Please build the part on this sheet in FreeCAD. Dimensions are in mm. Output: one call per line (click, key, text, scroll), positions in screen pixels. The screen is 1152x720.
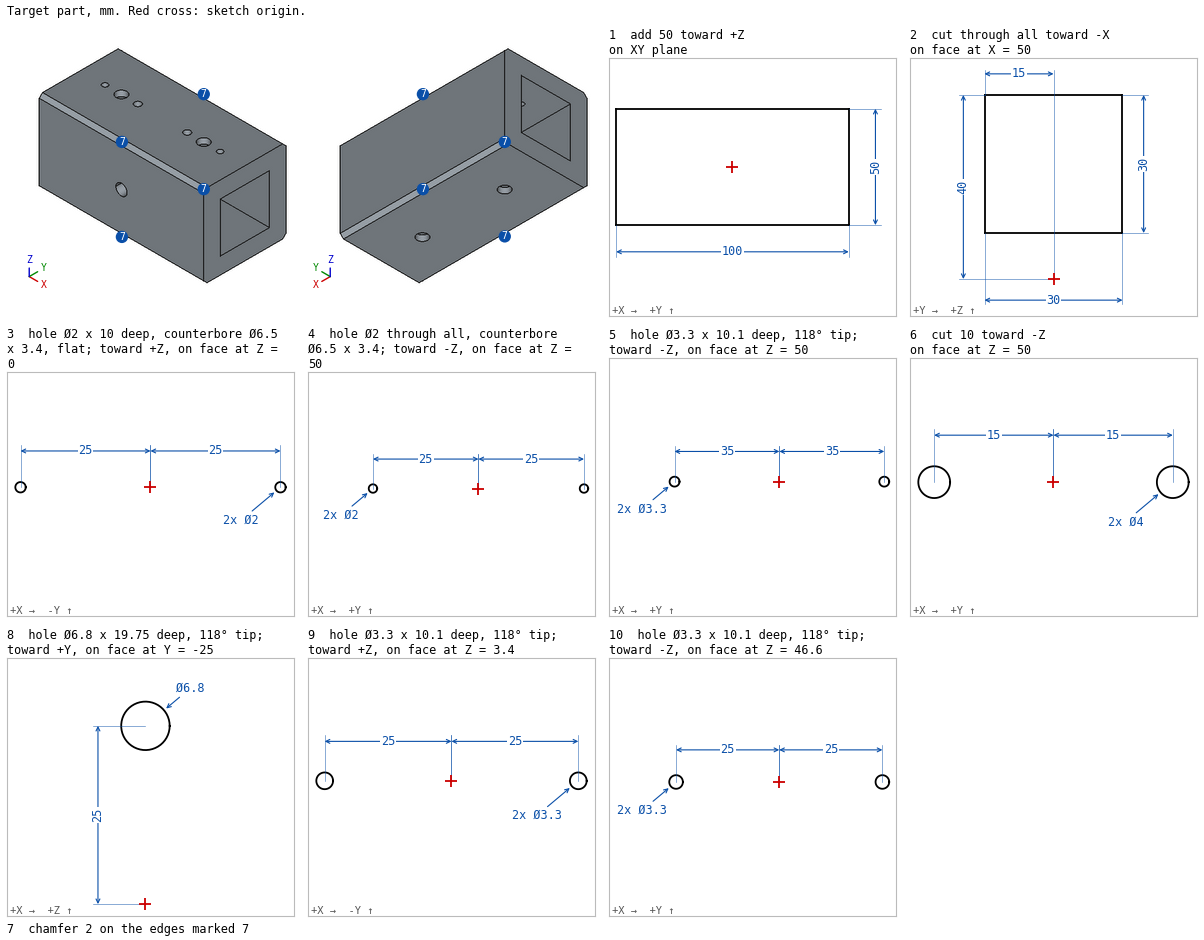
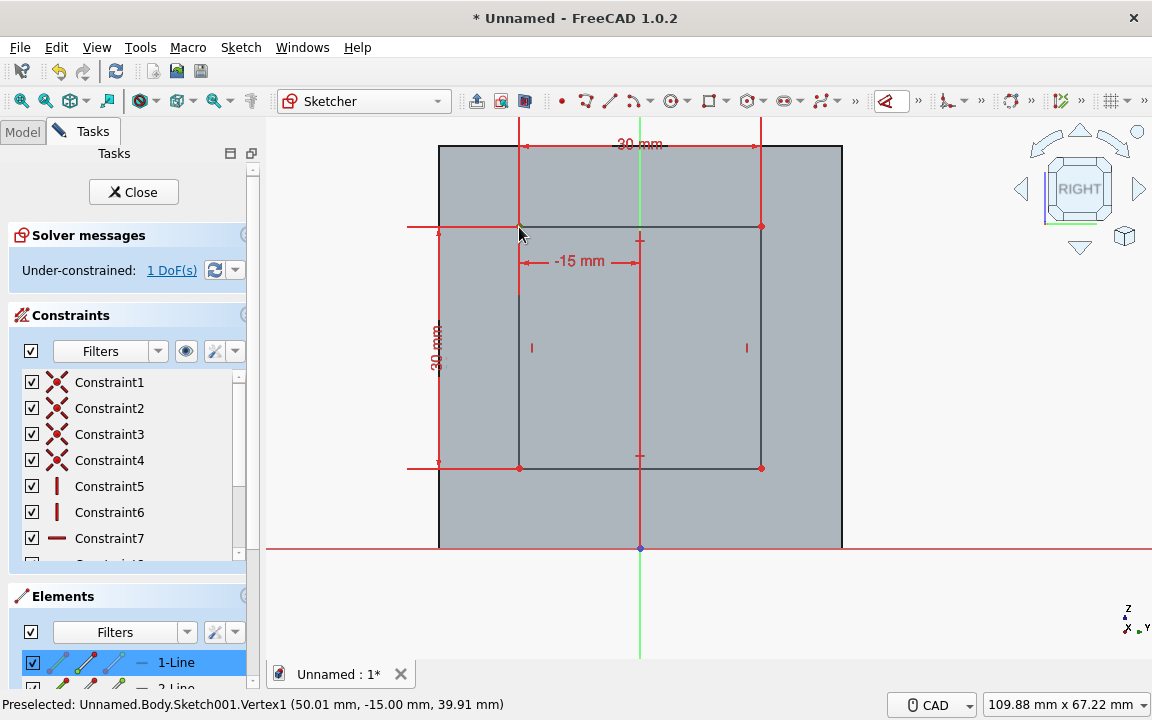
click(904, 102)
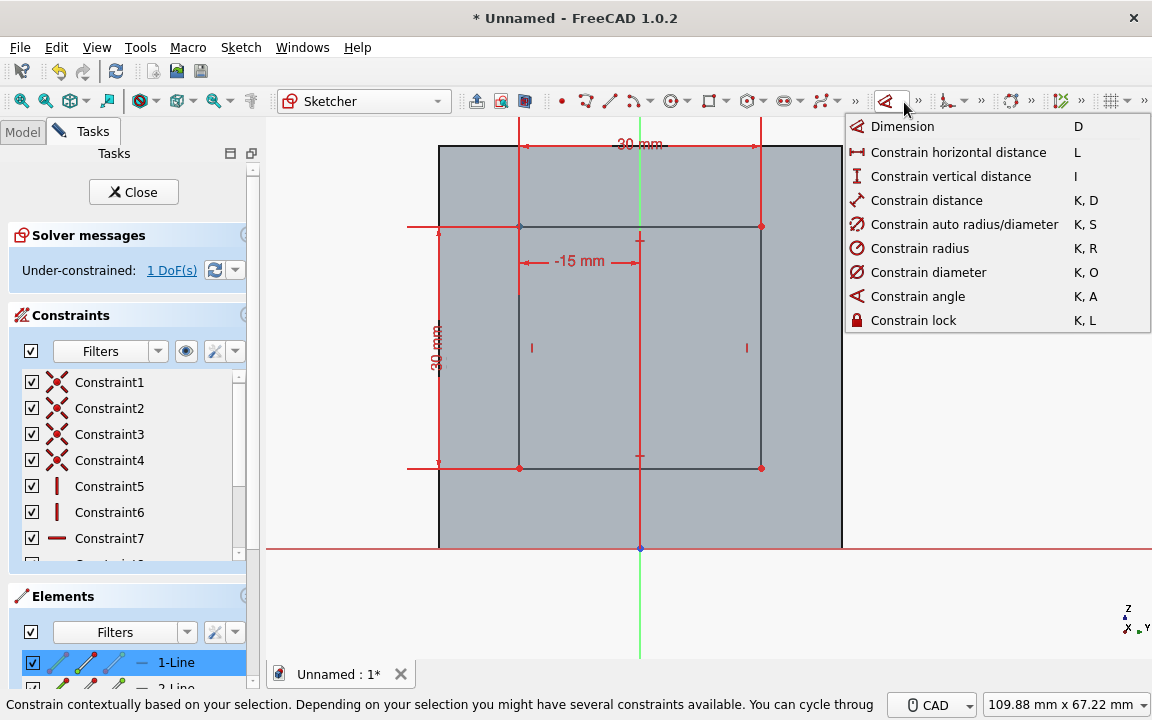
click(998, 176)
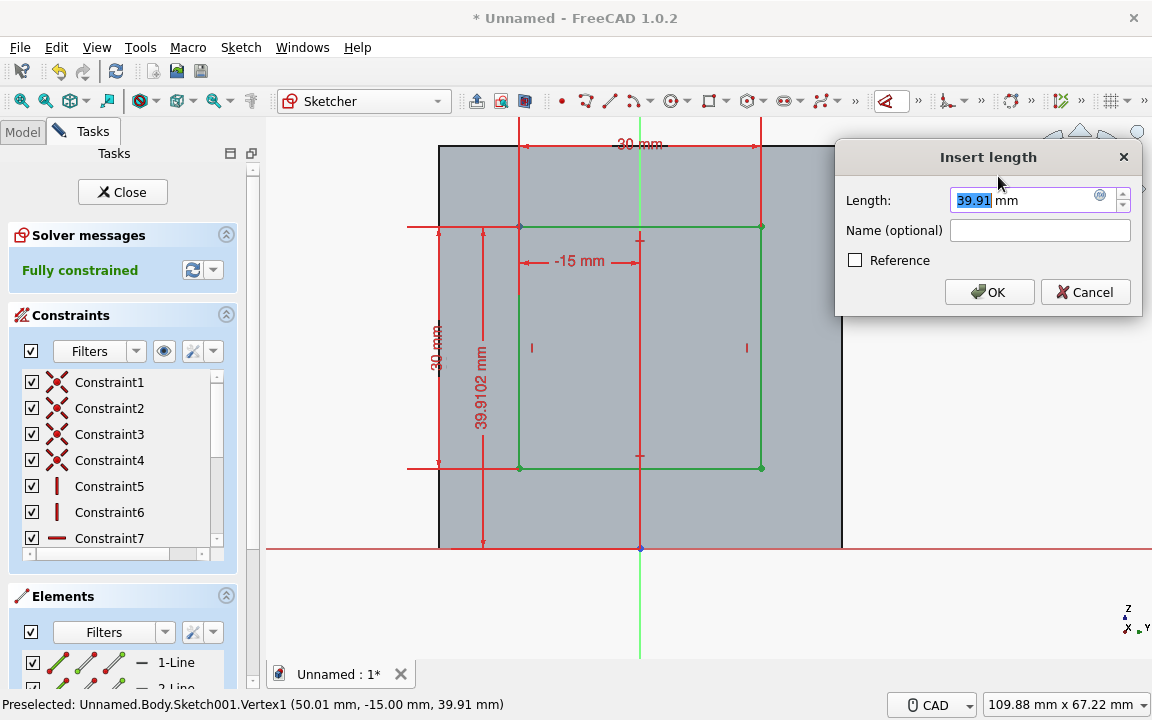
text(40)
key(Return)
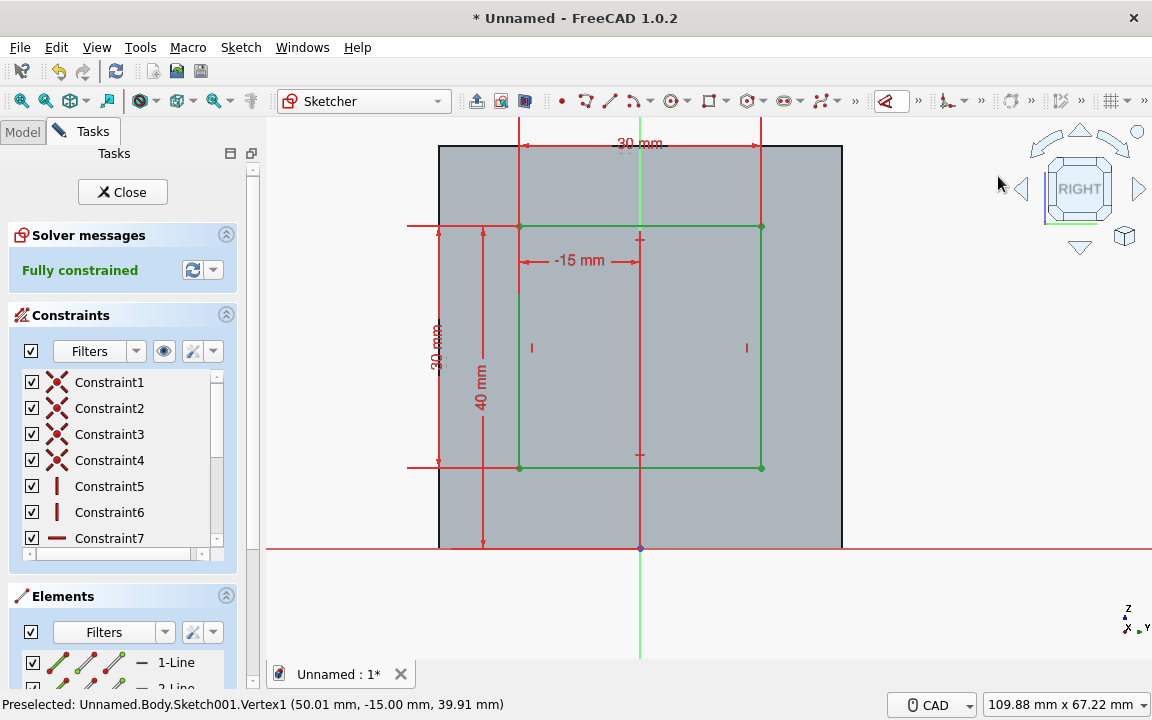
click(123, 192)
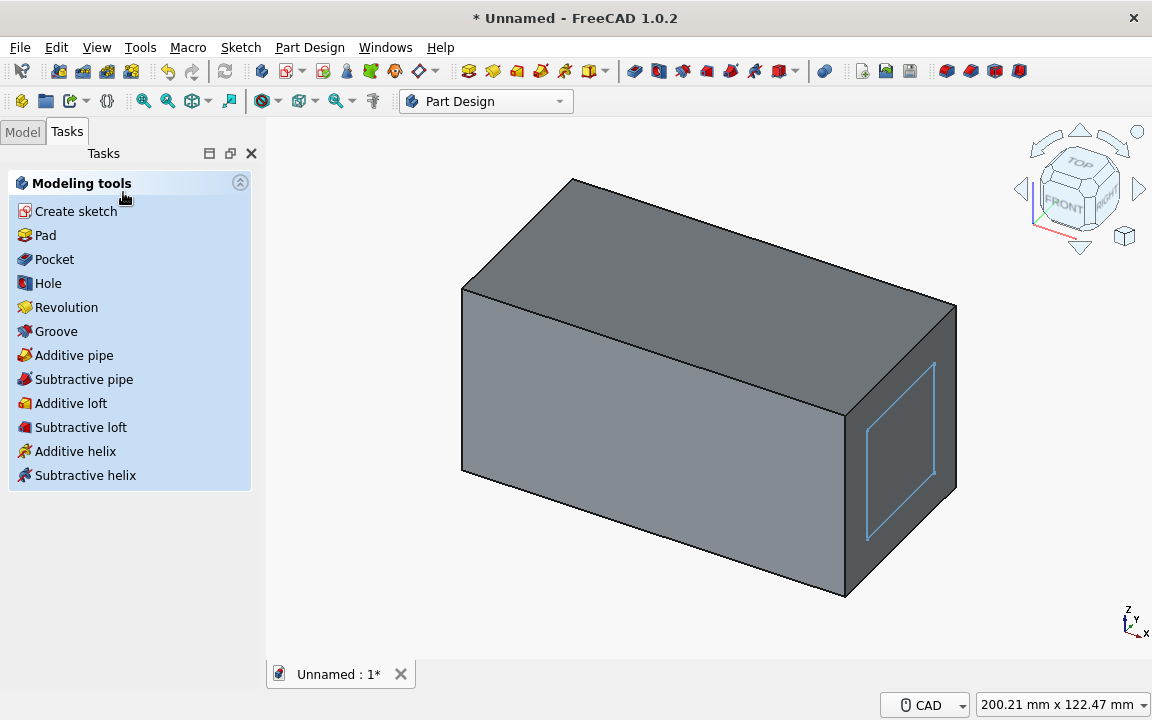
click(636, 72)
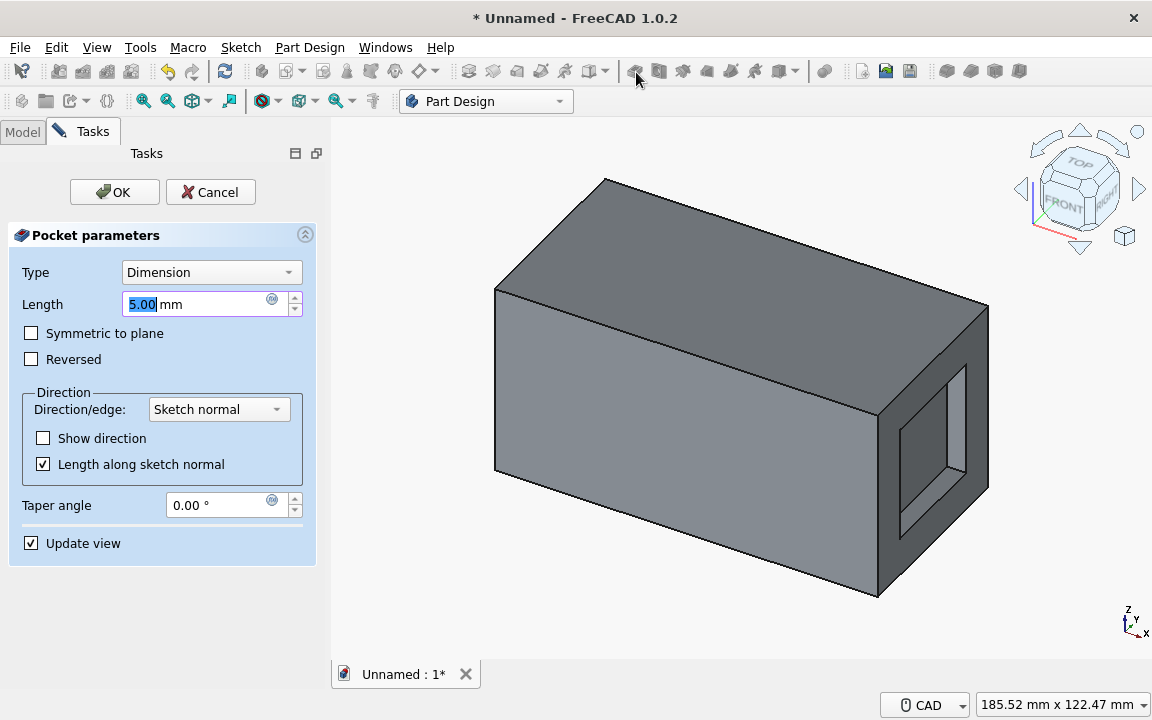
click(212, 272)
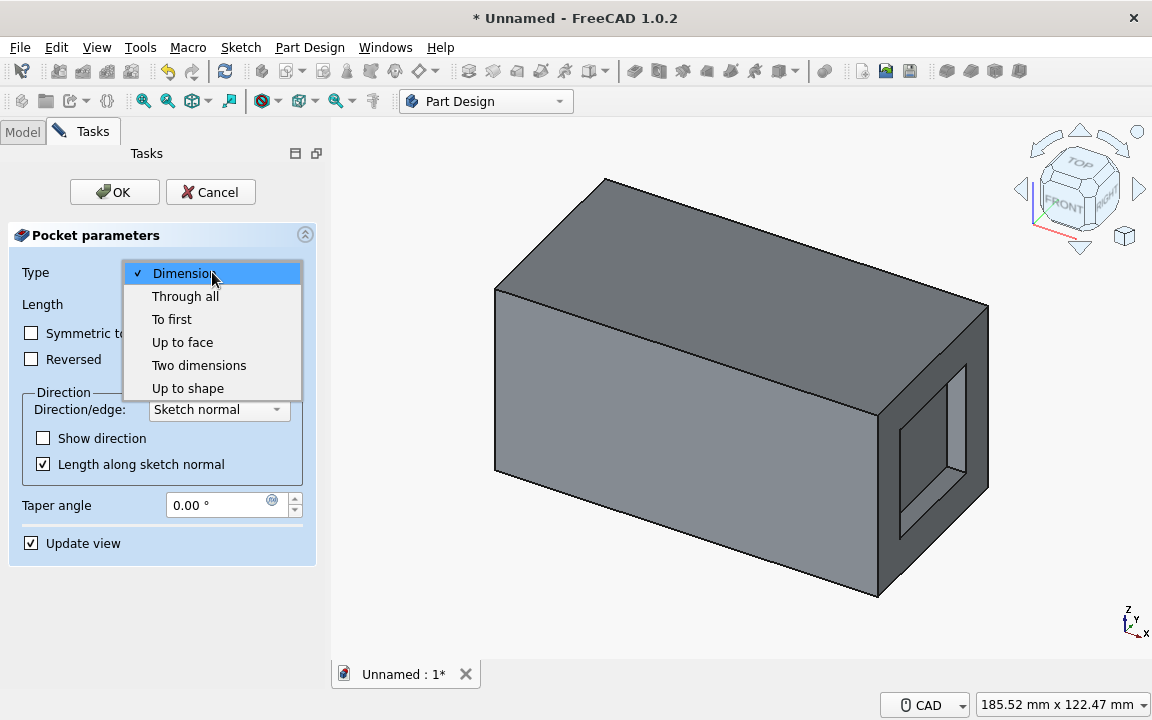
click(212, 296)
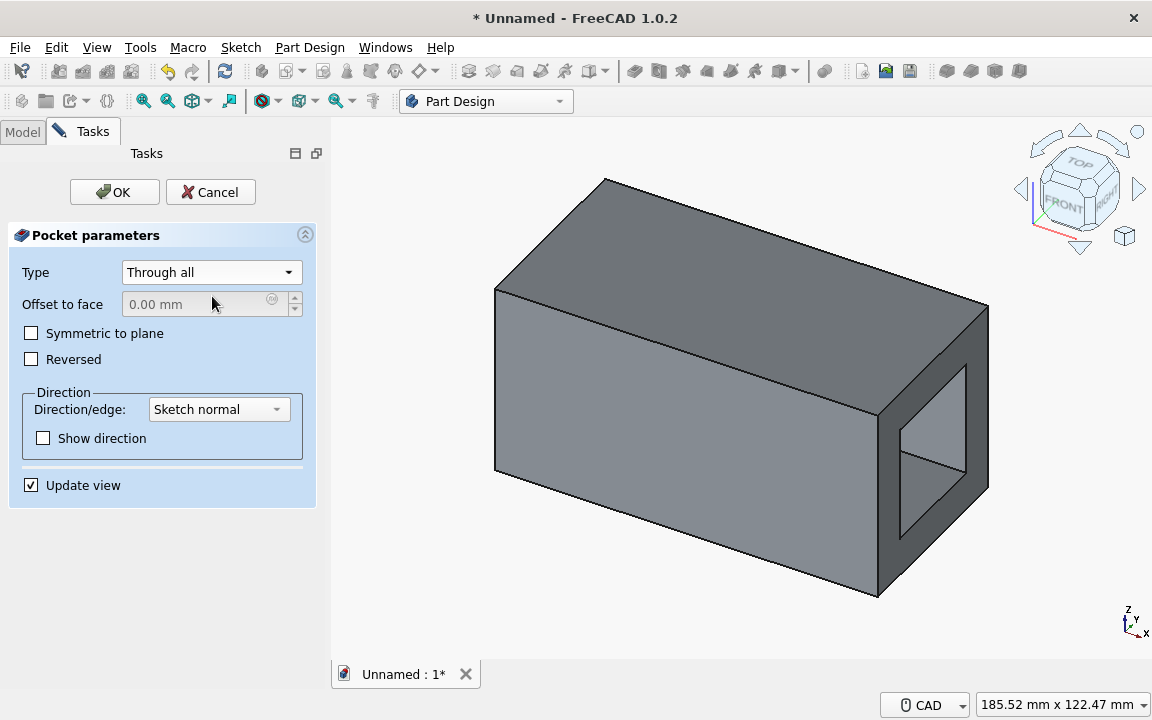
click(115, 192)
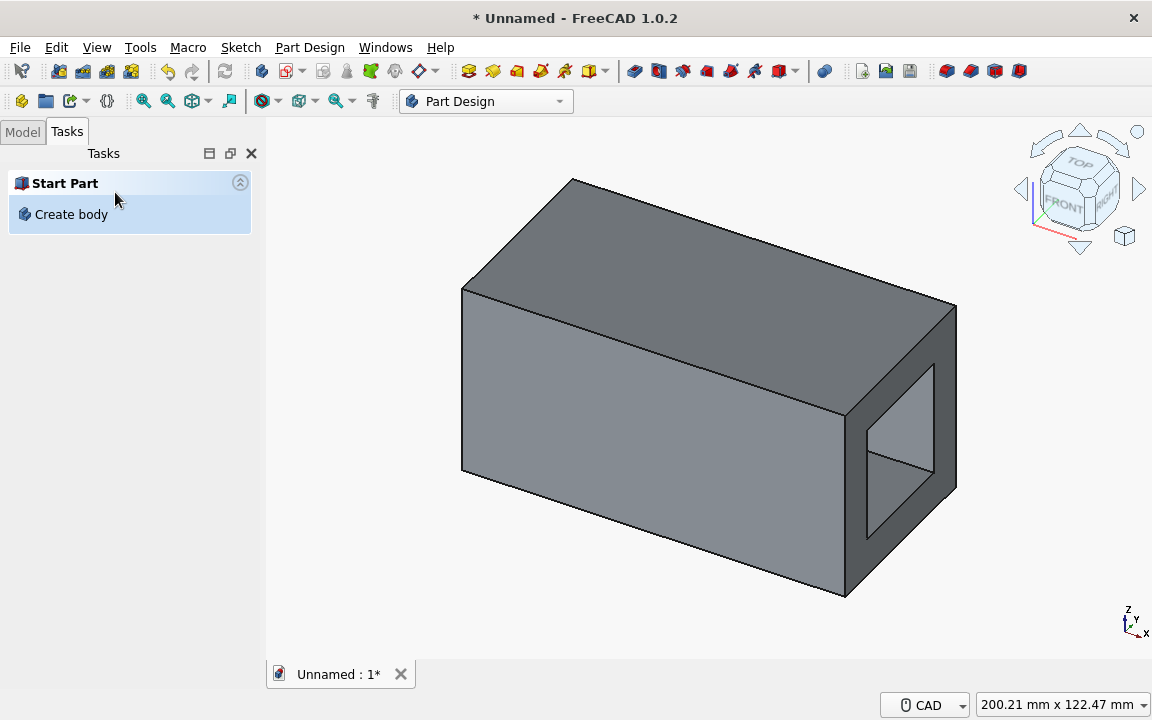
key(5)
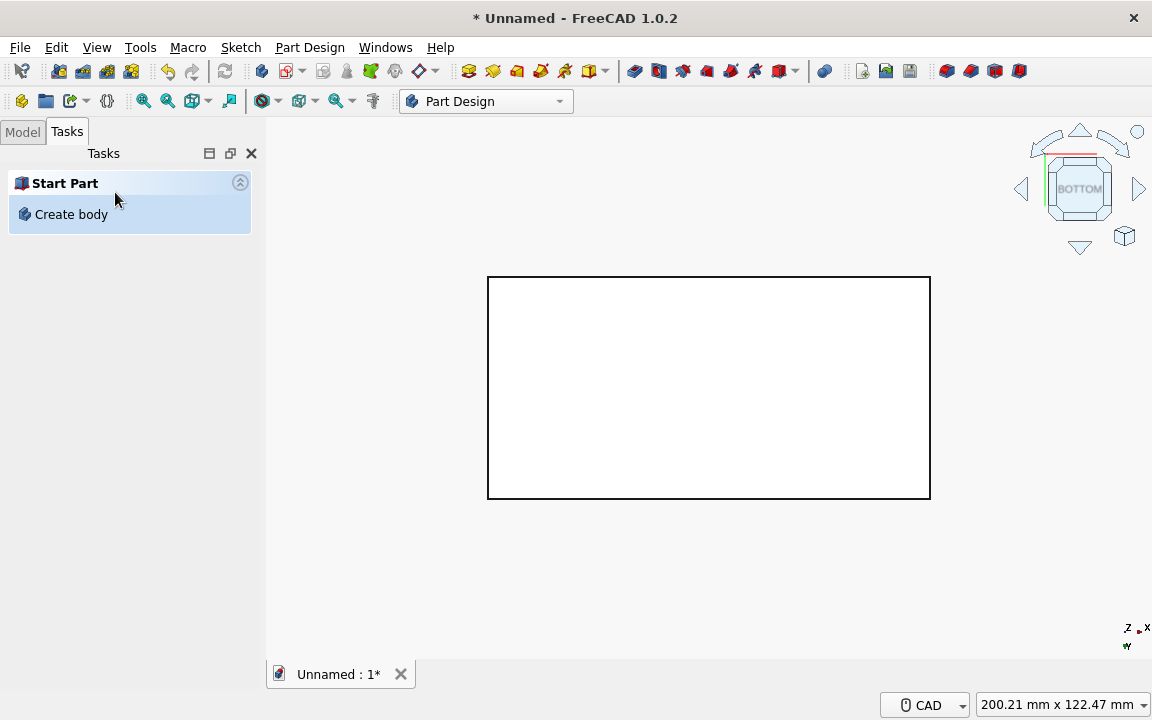
click(772, 387)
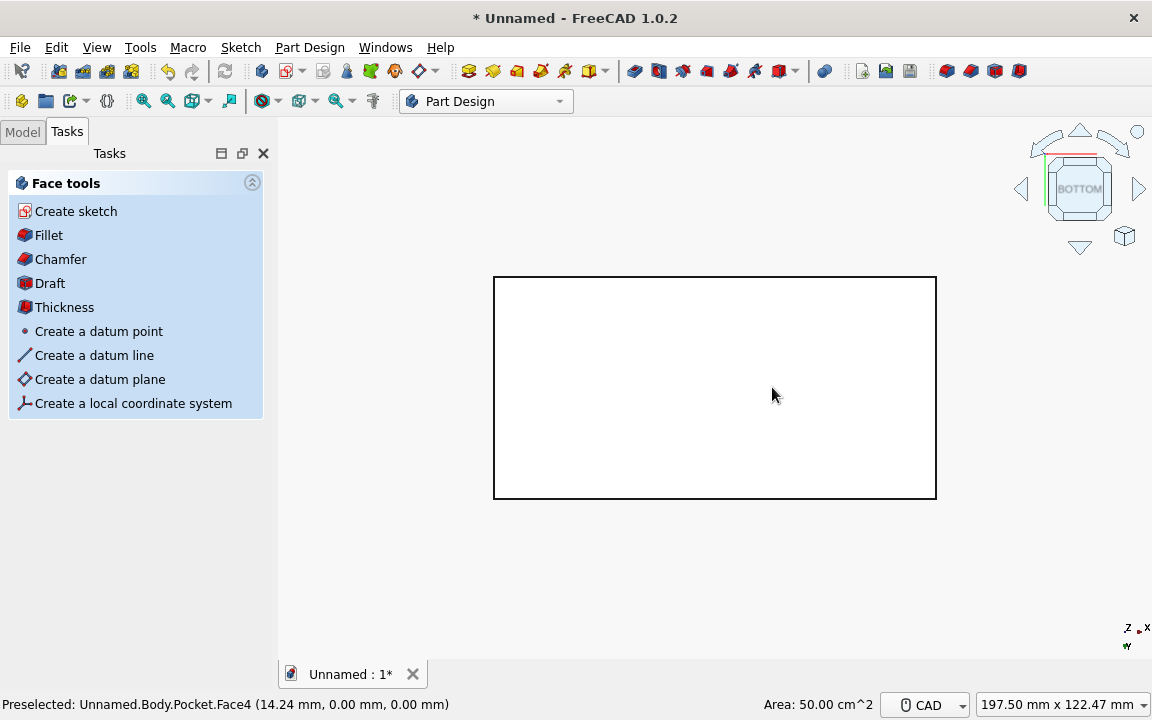
click(286, 72)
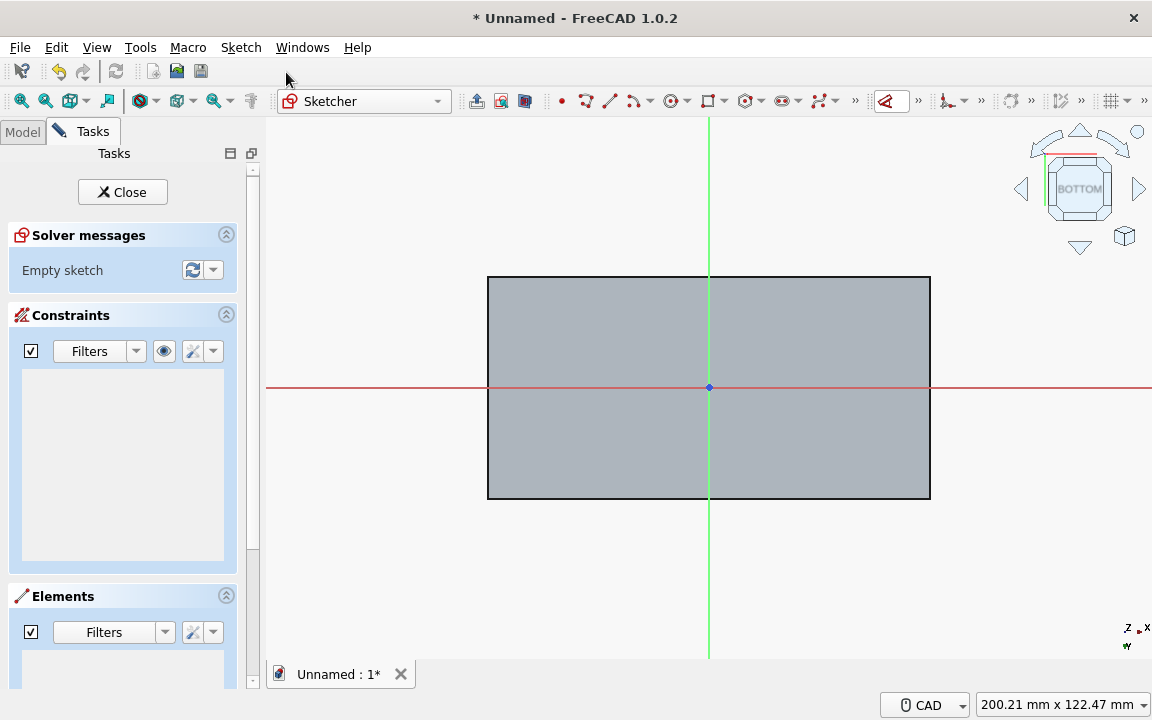
scroll(765, 388, up, 4)